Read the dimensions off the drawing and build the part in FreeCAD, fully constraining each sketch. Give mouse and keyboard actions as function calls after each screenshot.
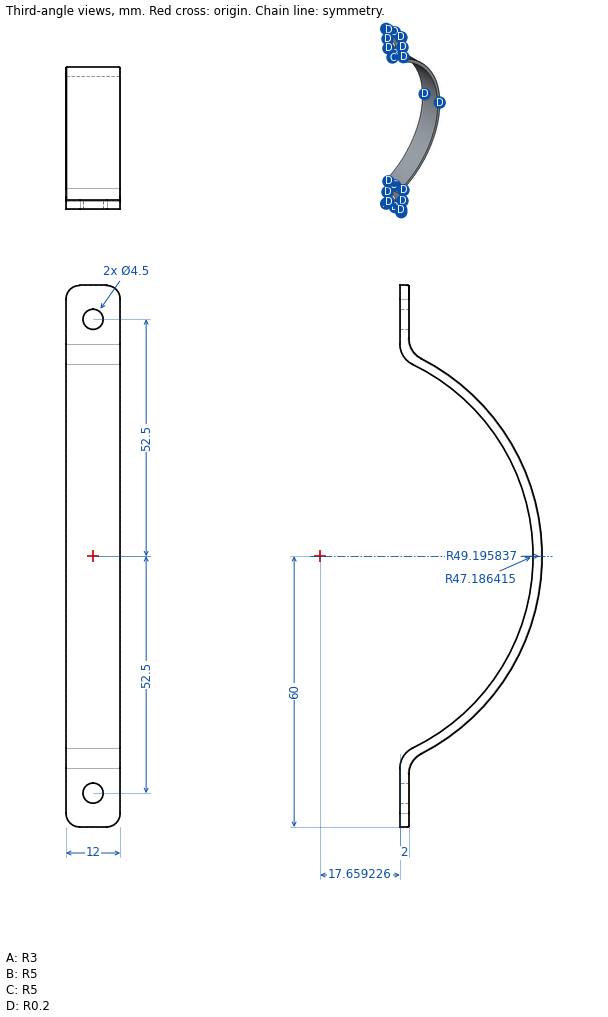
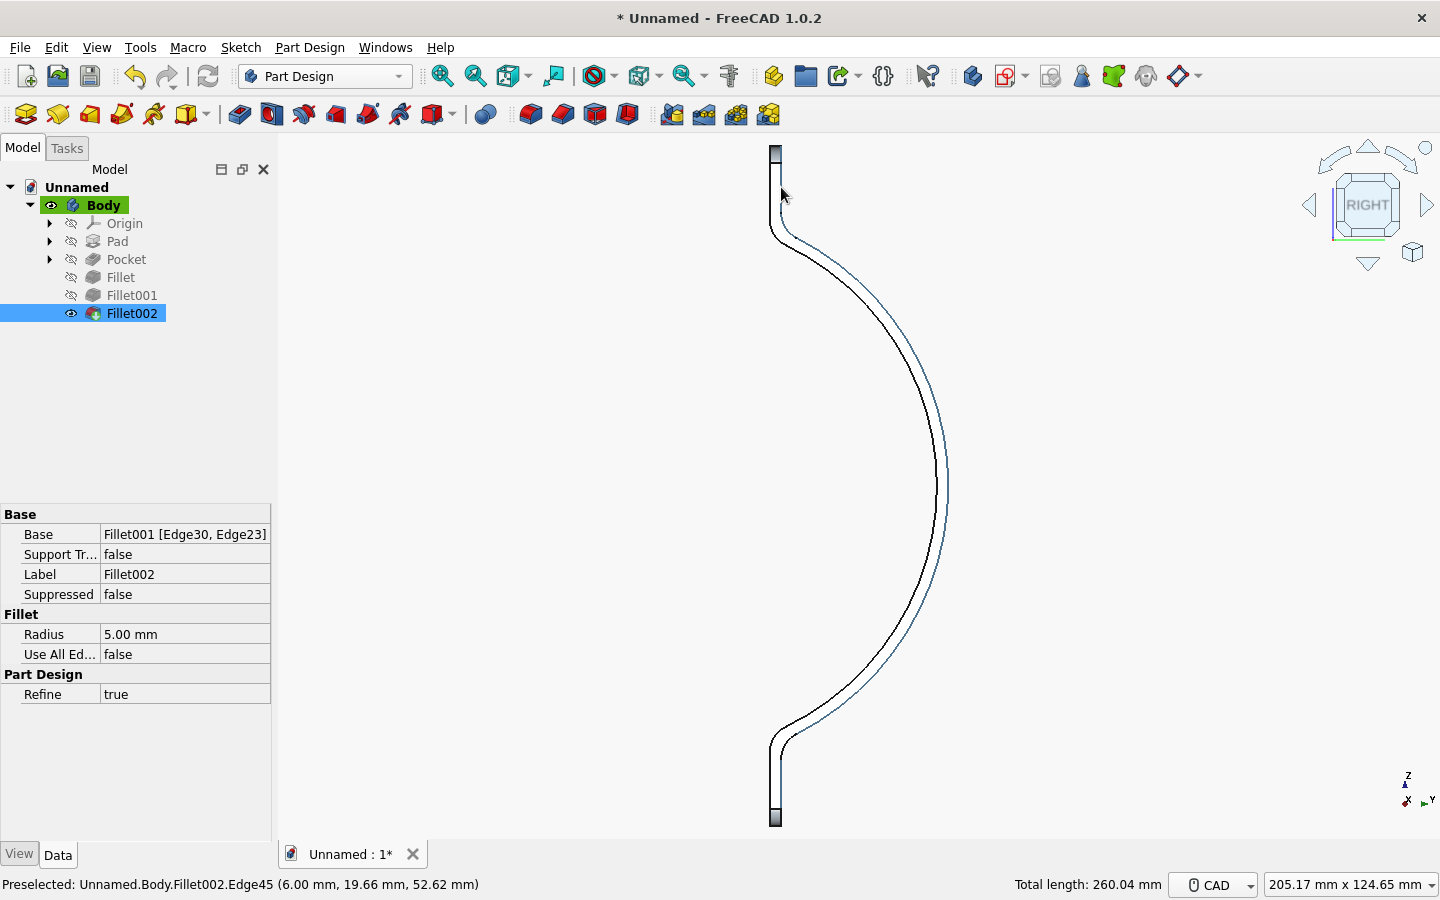
click(785, 744, ctrl)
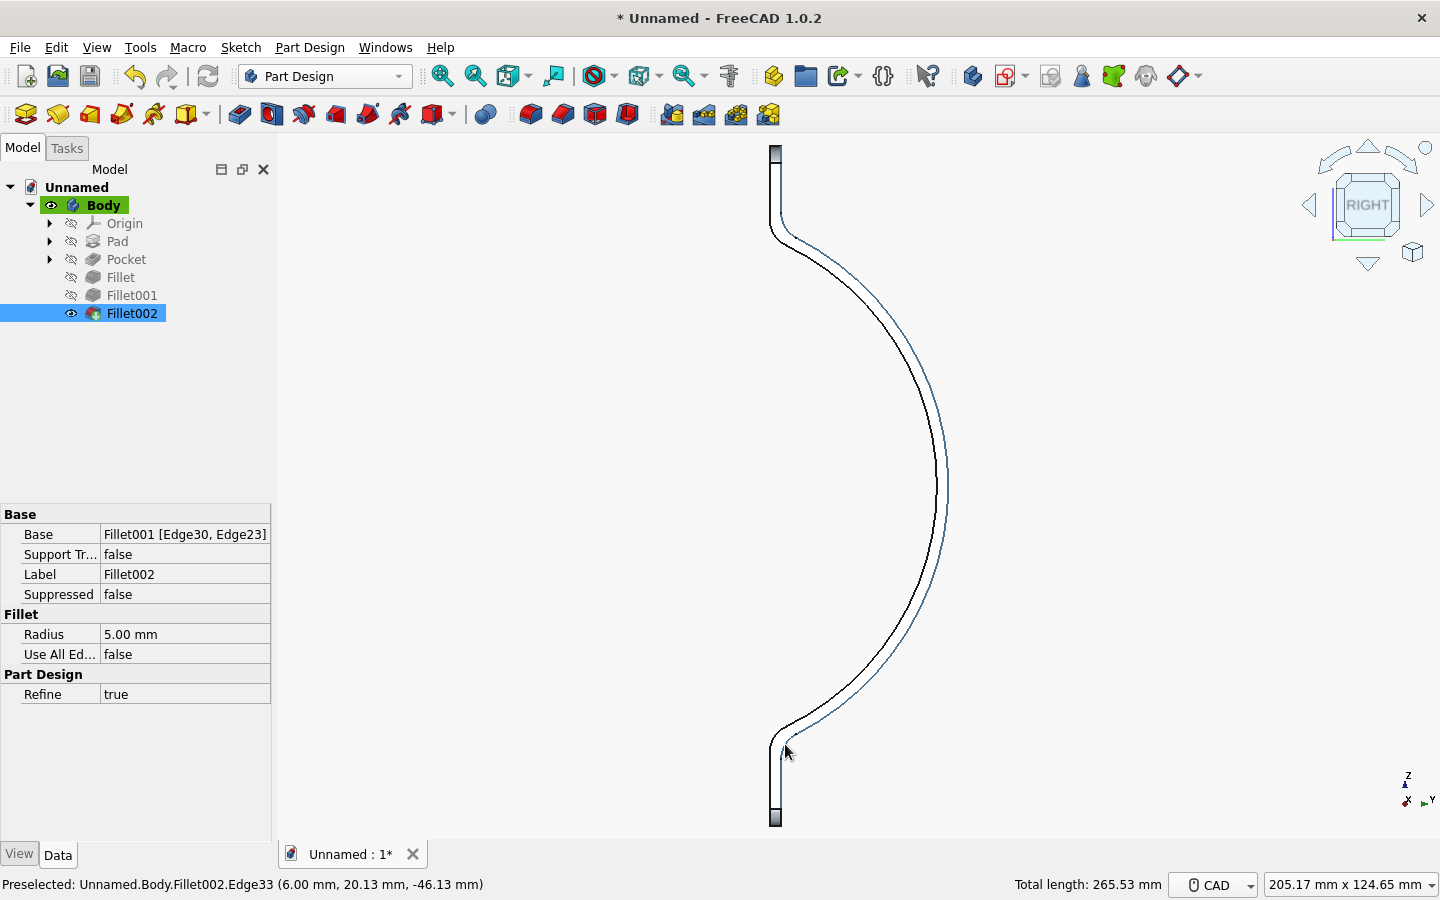
key(5)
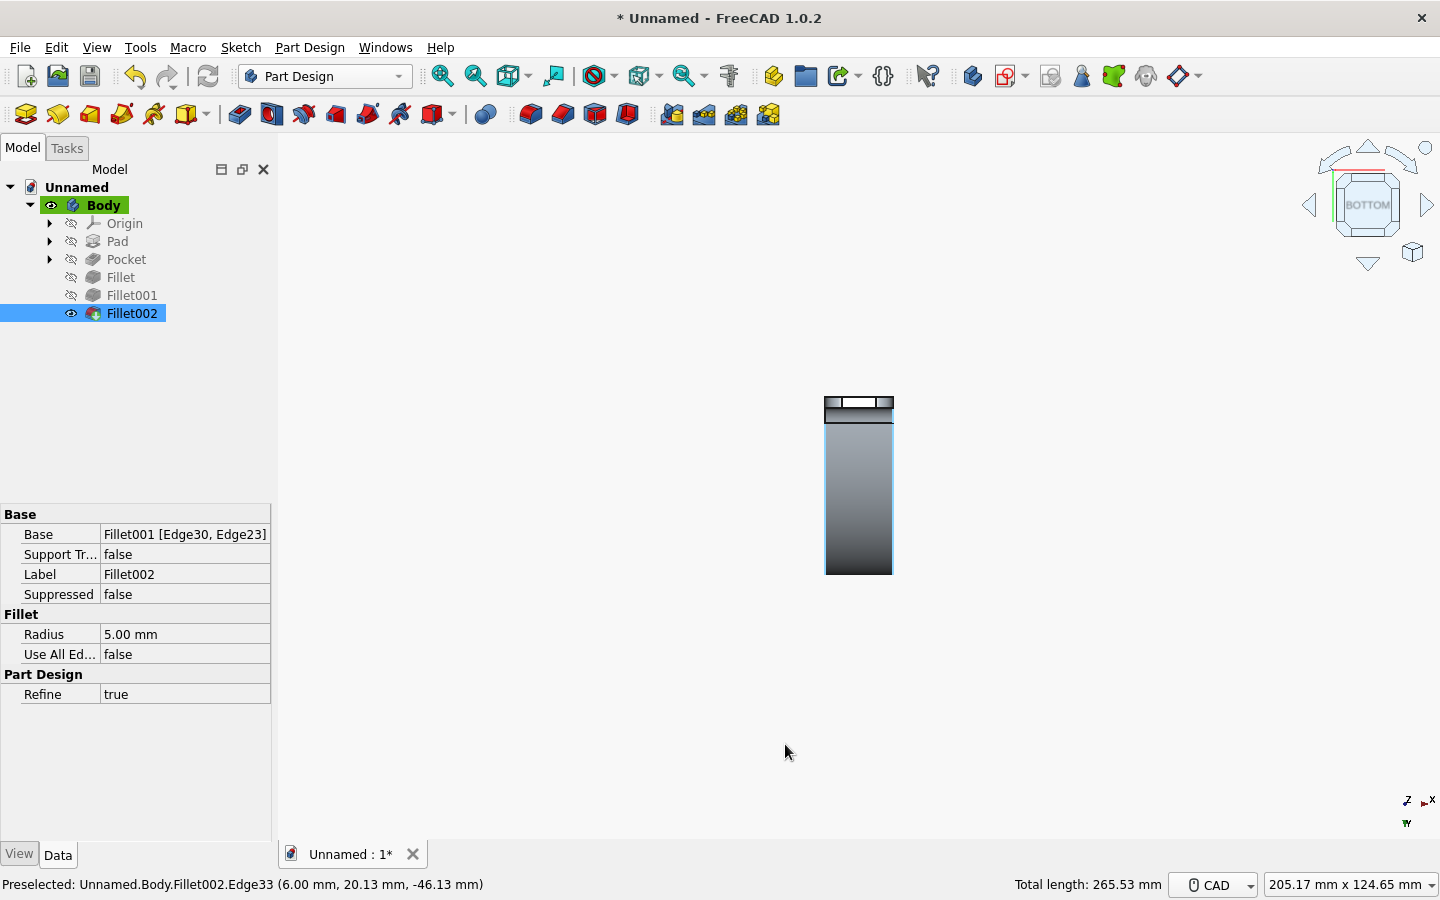
click(444, 76)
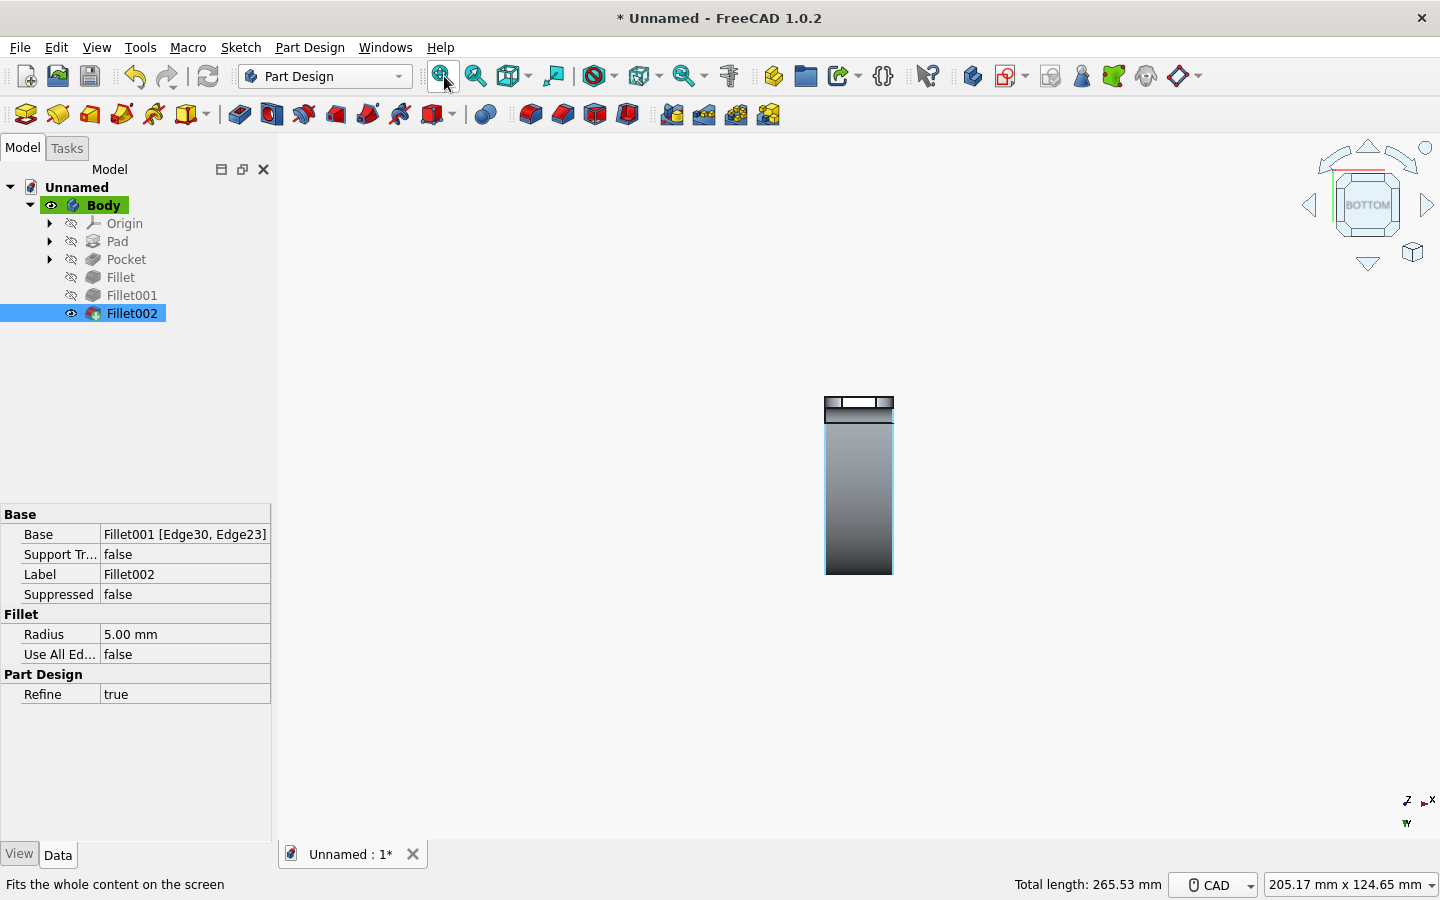
click(859, 407, ctrl)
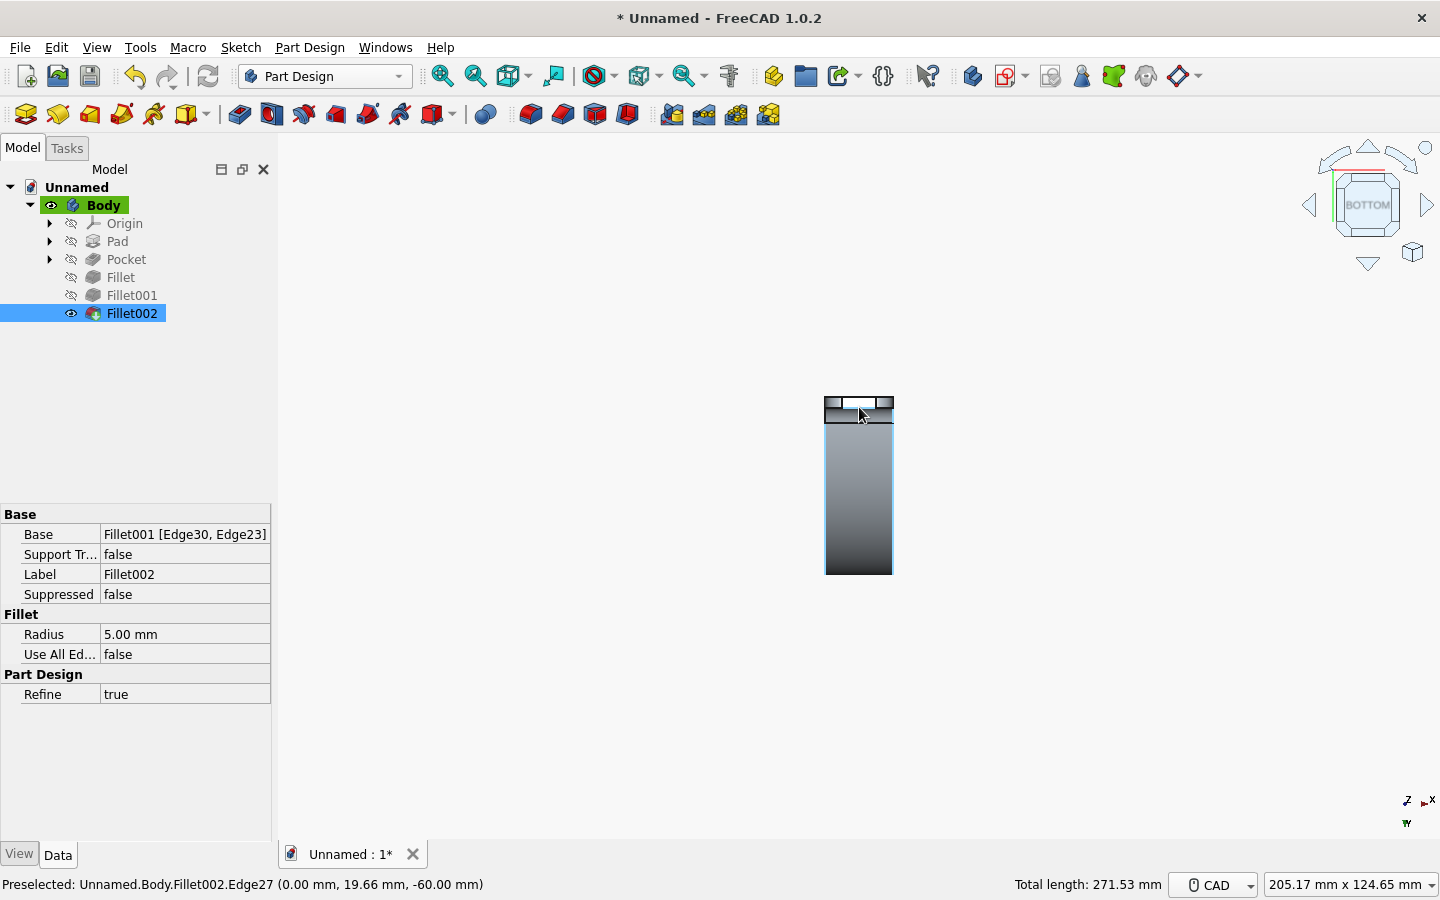
click(888, 407, ctrl)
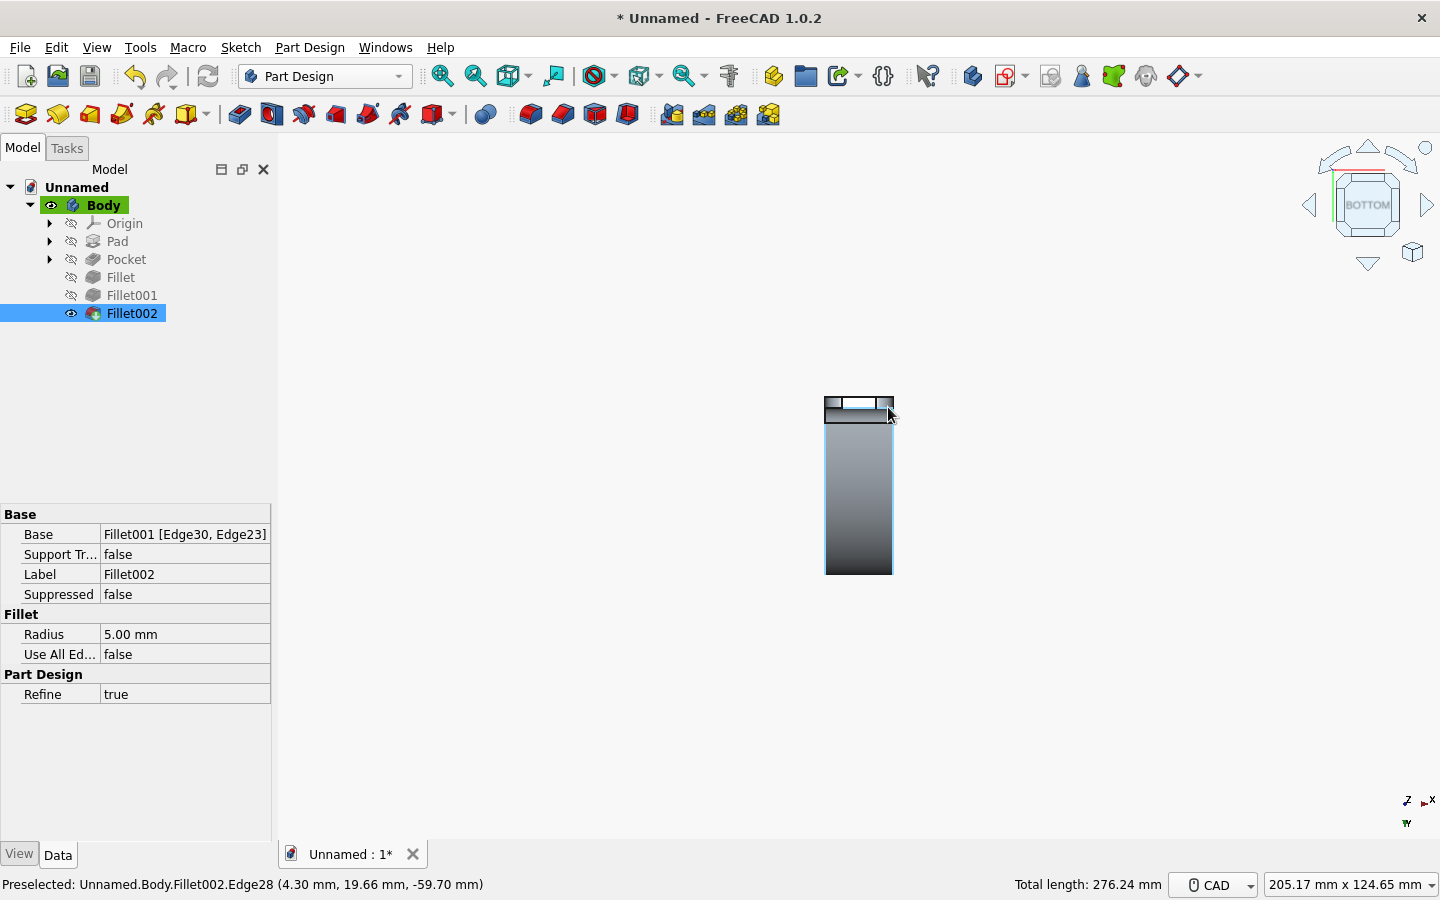
click(830, 407, ctrl)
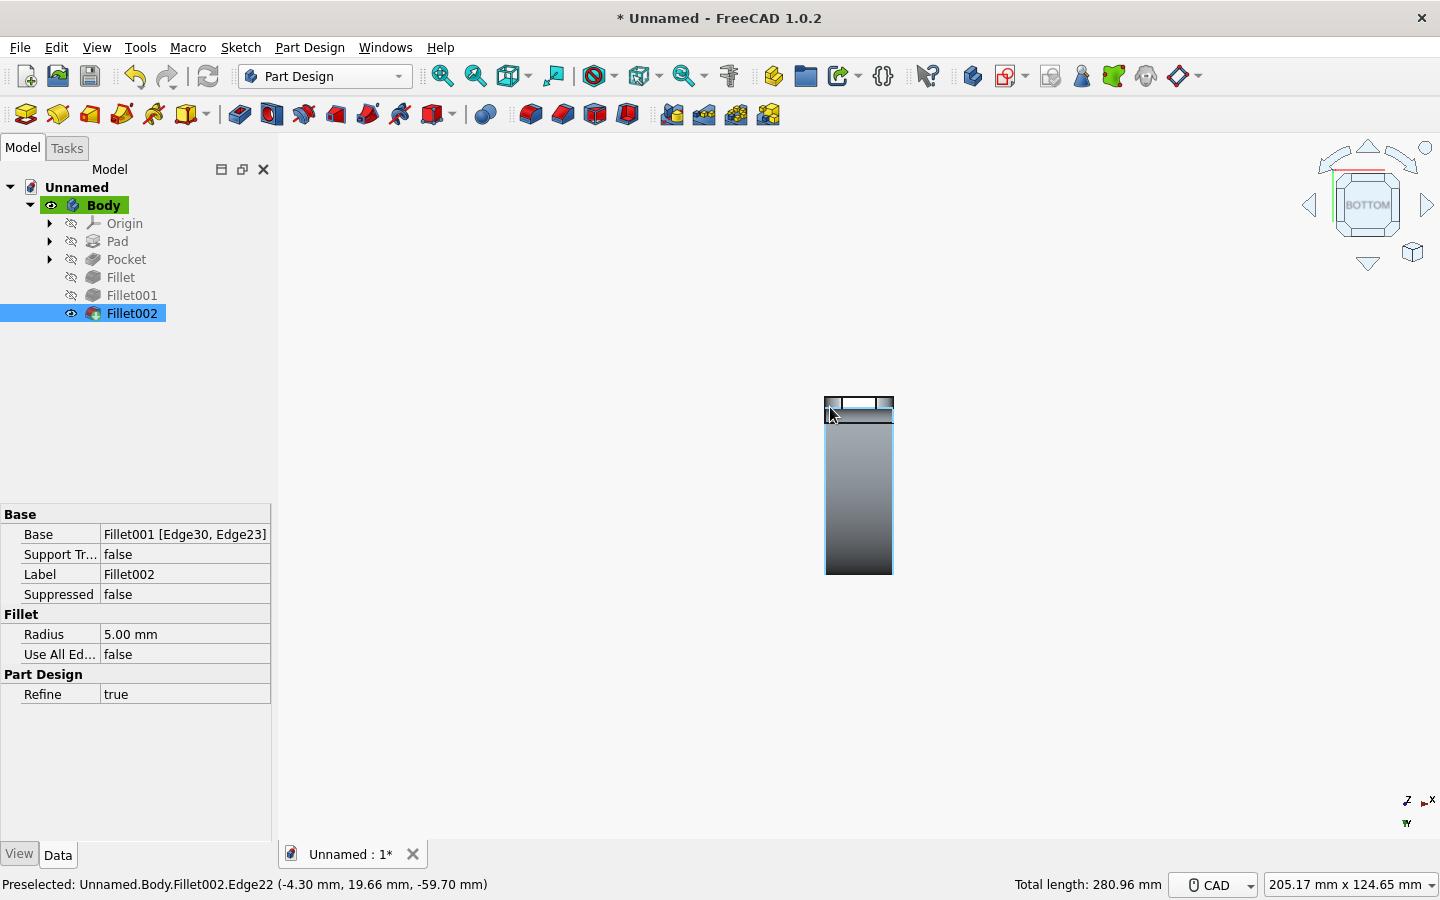
click(825, 415, ctrl)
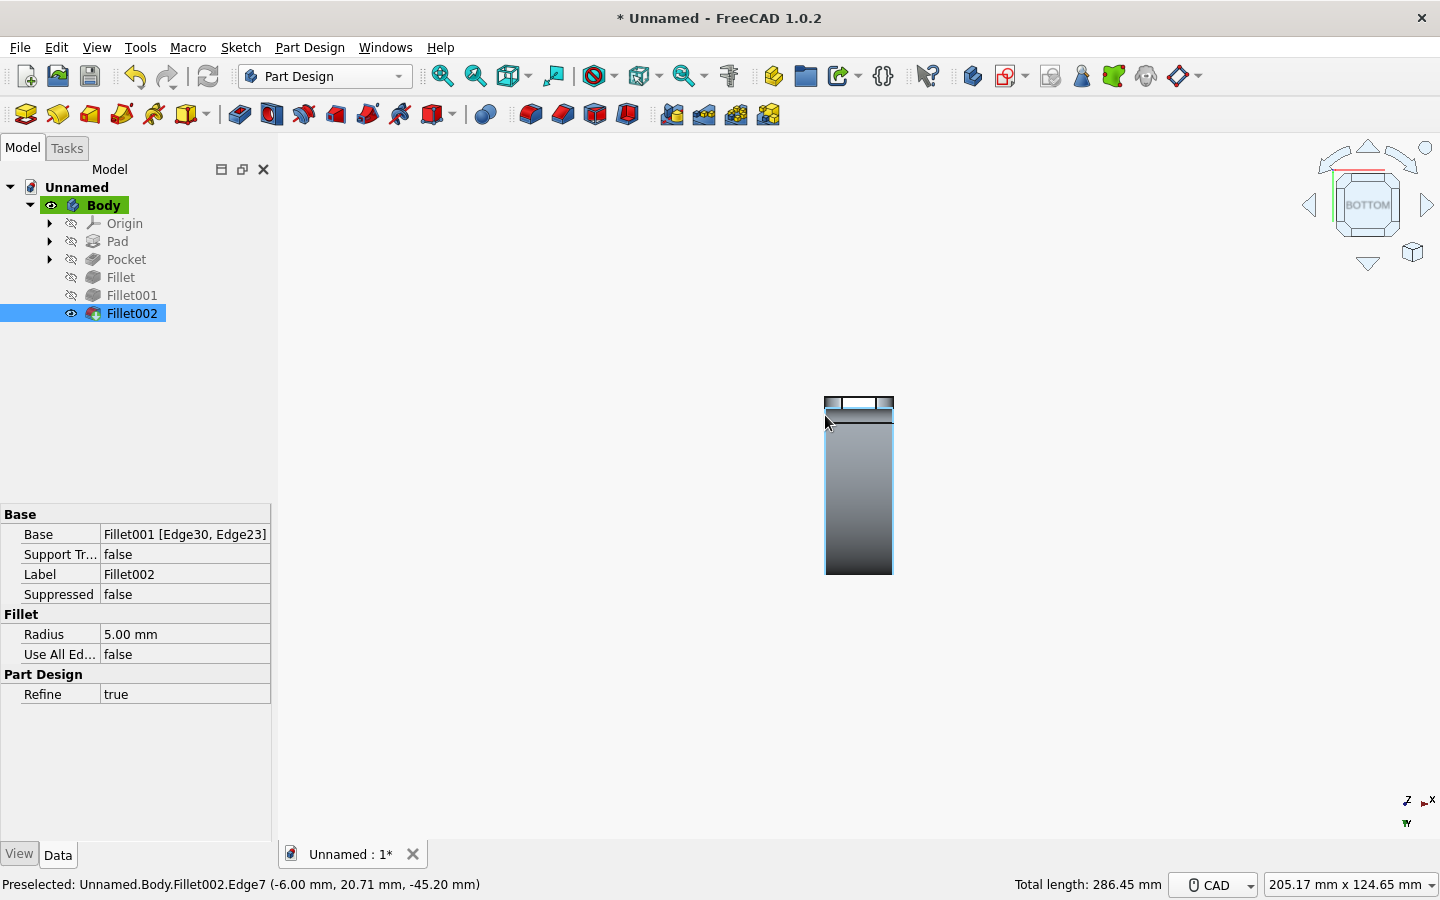
key(4)